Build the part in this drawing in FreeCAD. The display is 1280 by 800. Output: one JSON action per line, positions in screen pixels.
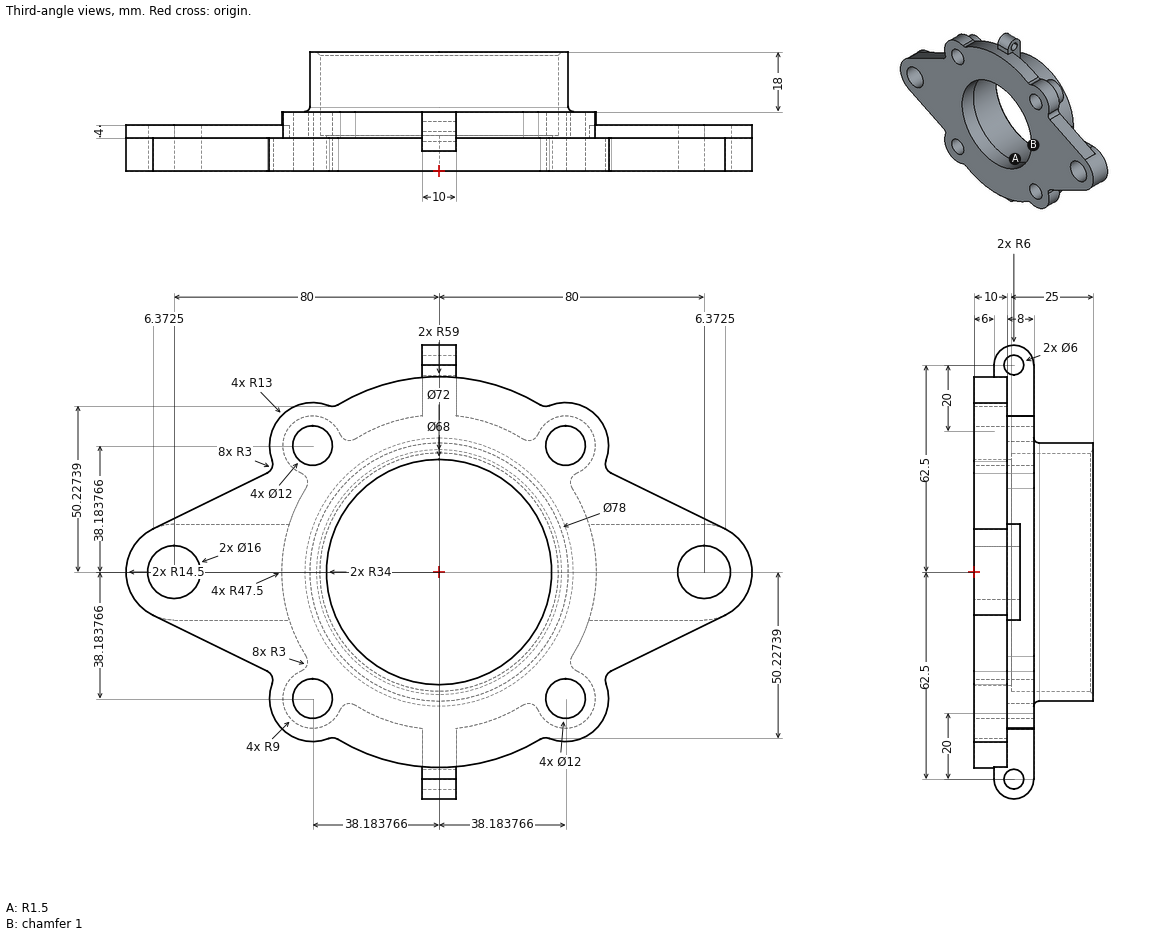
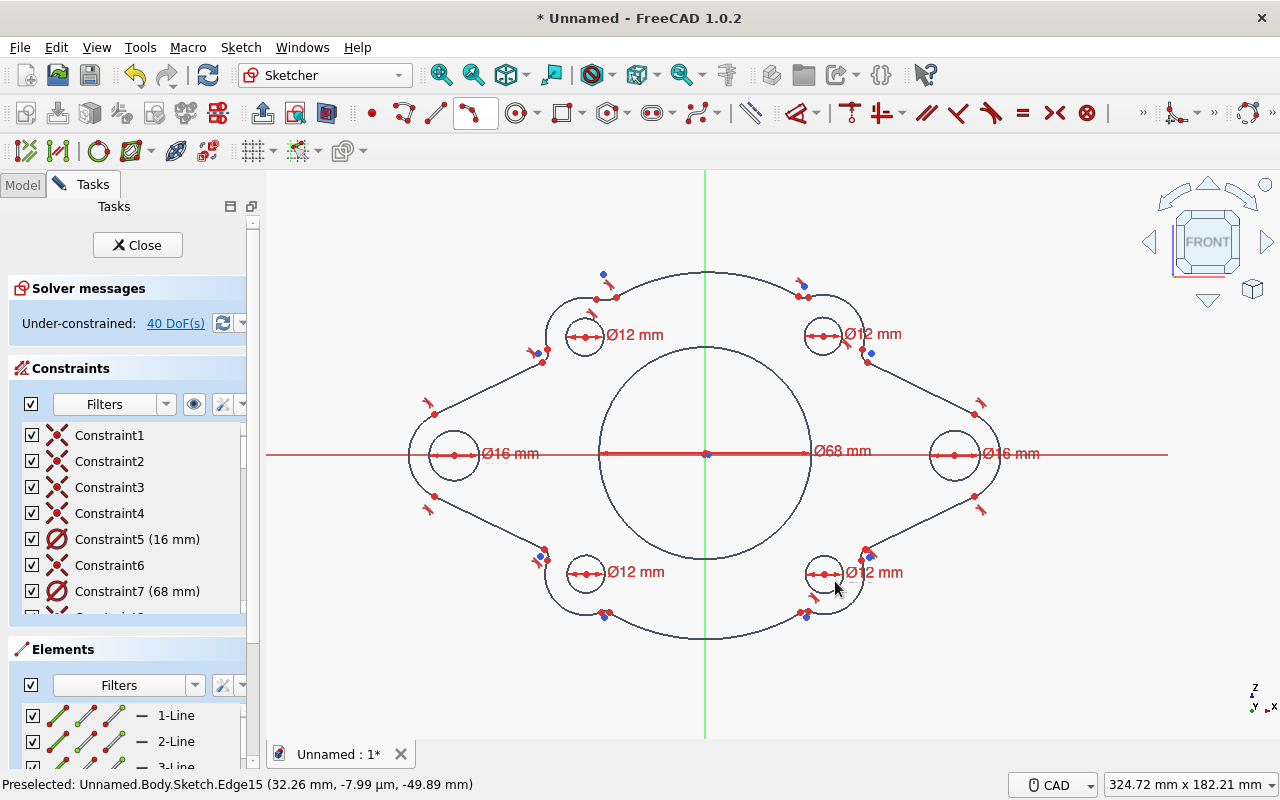
{"action": "left_click", "coordinate": [665, 635]}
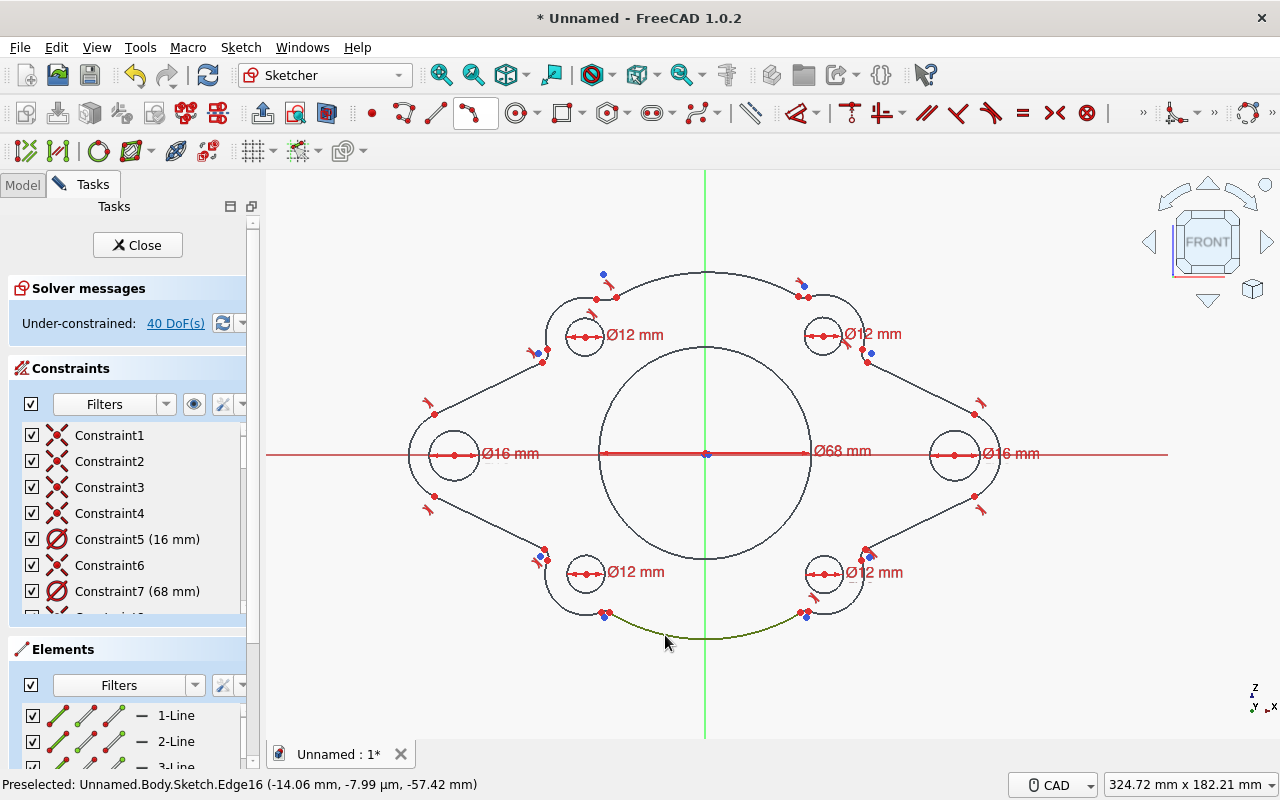
{"action": "left_click", "coordinate": [992, 114]}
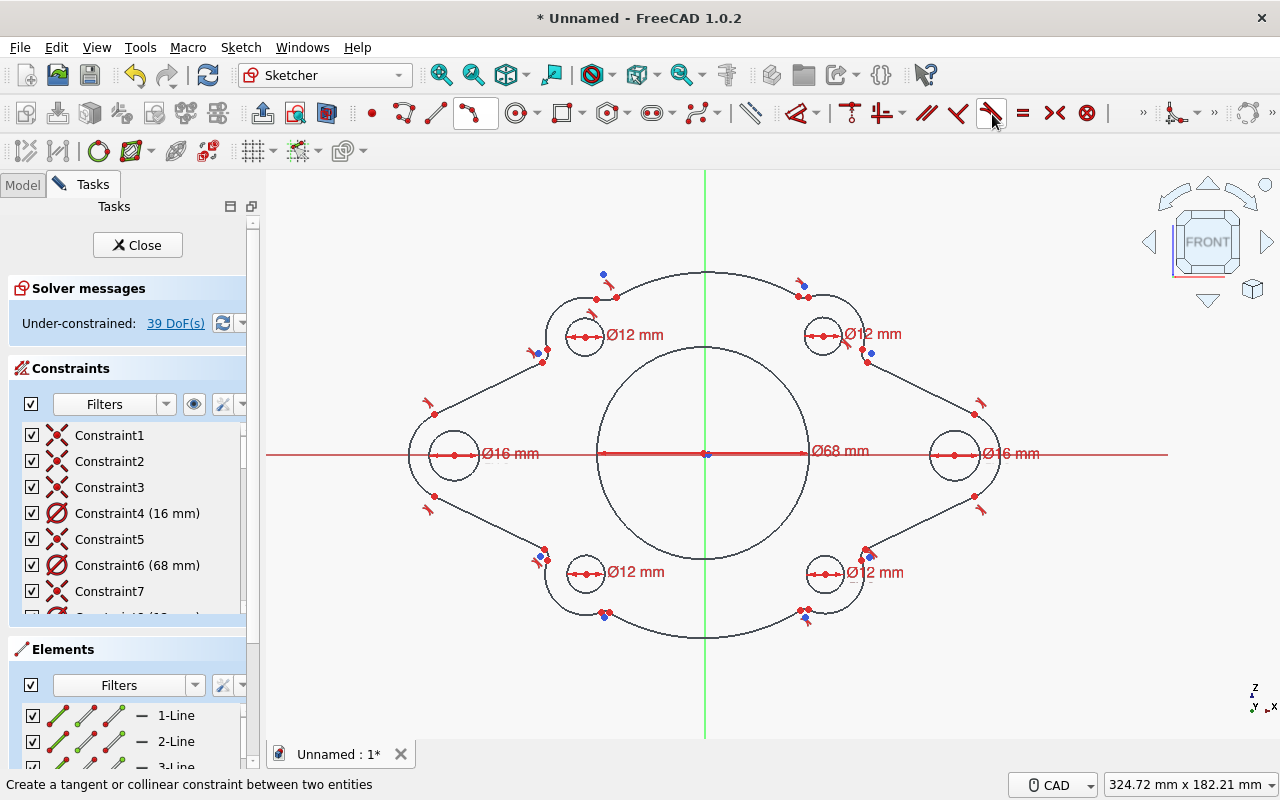
{"action": "left_click", "coordinate": [665, 634]}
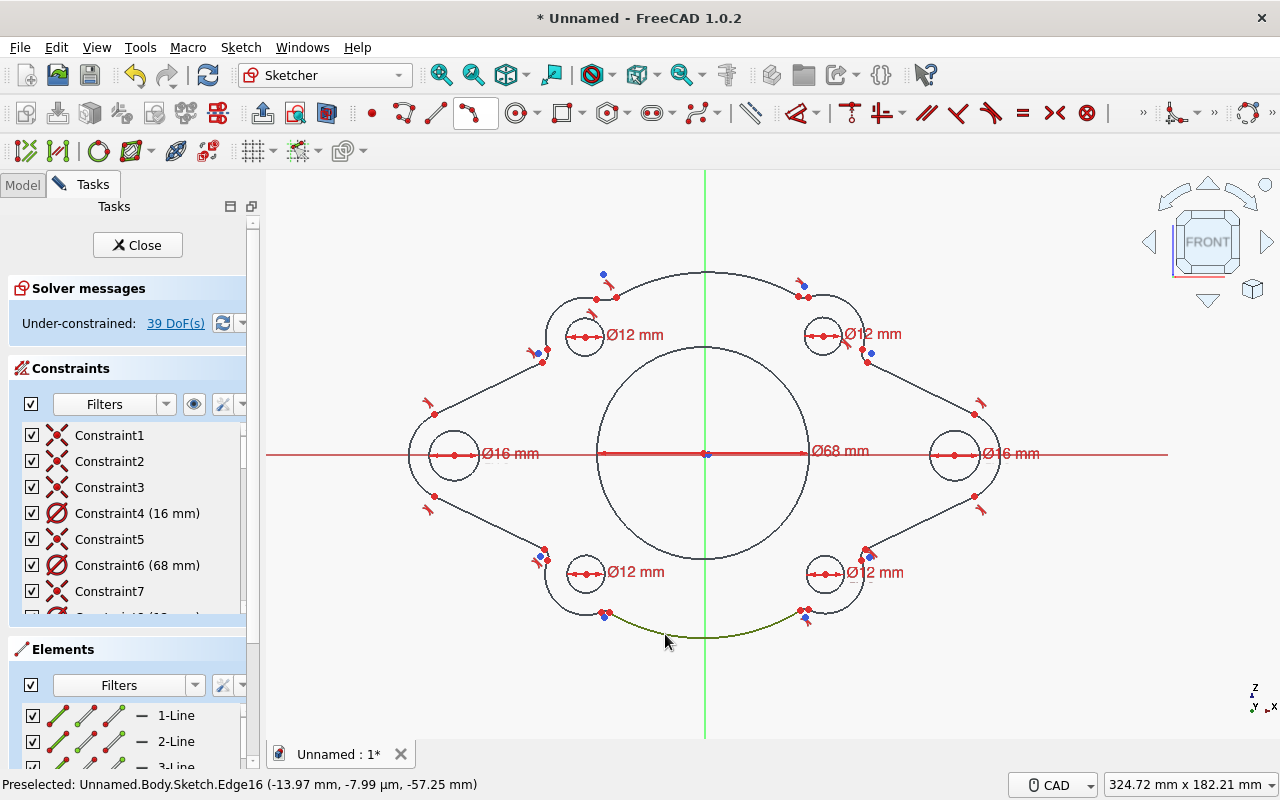
{"action": "scroll", "coordinate": [605, 611], "scroll_direction": "up", "scroll_amount": 6}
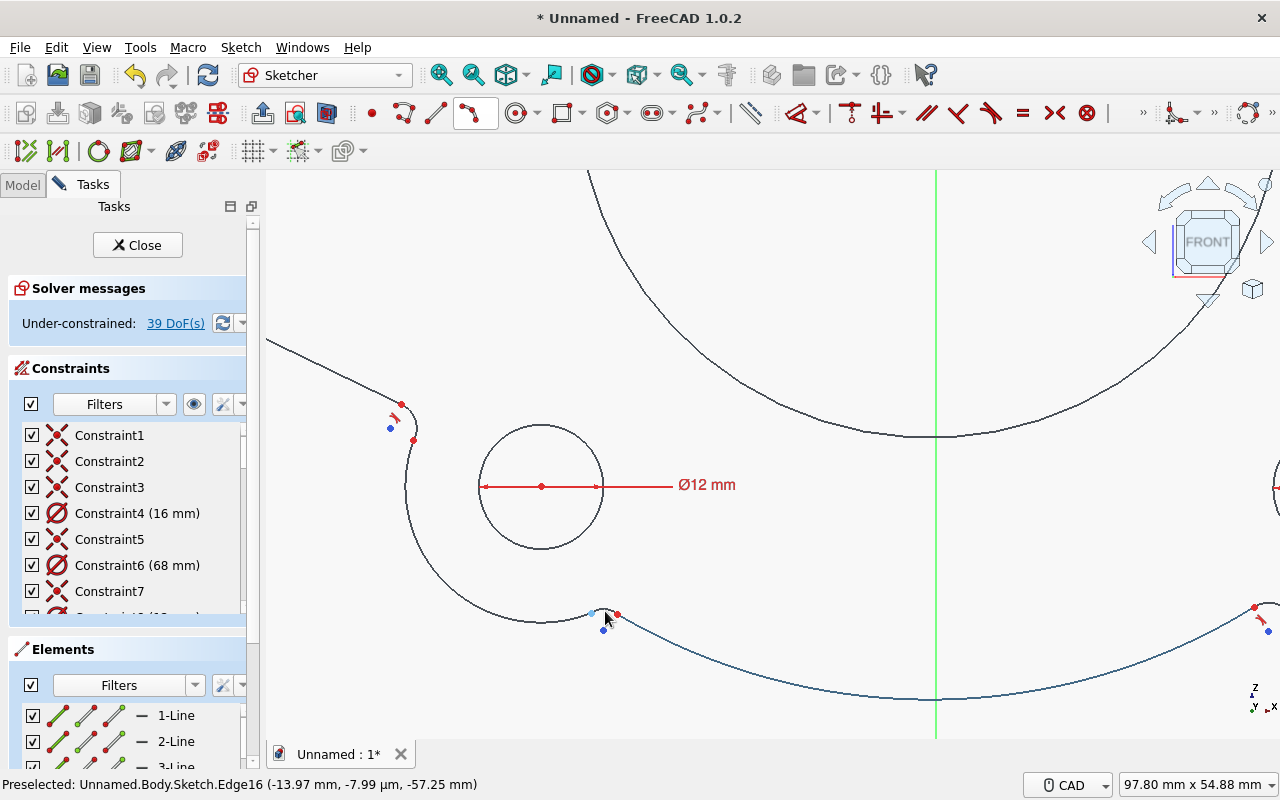
{"action": "left_click", "coordinate": [605, 609]}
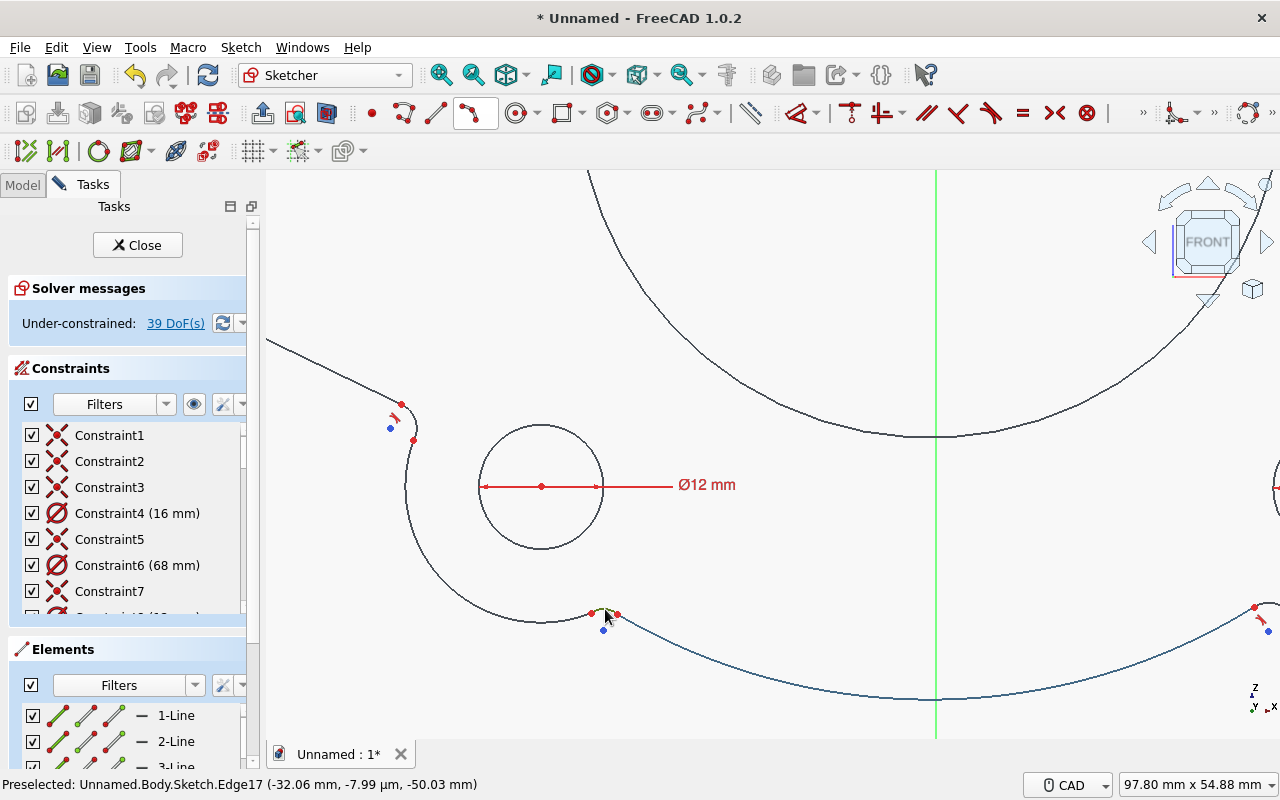
{"action": "left_click", "coordinate": [992, 114]}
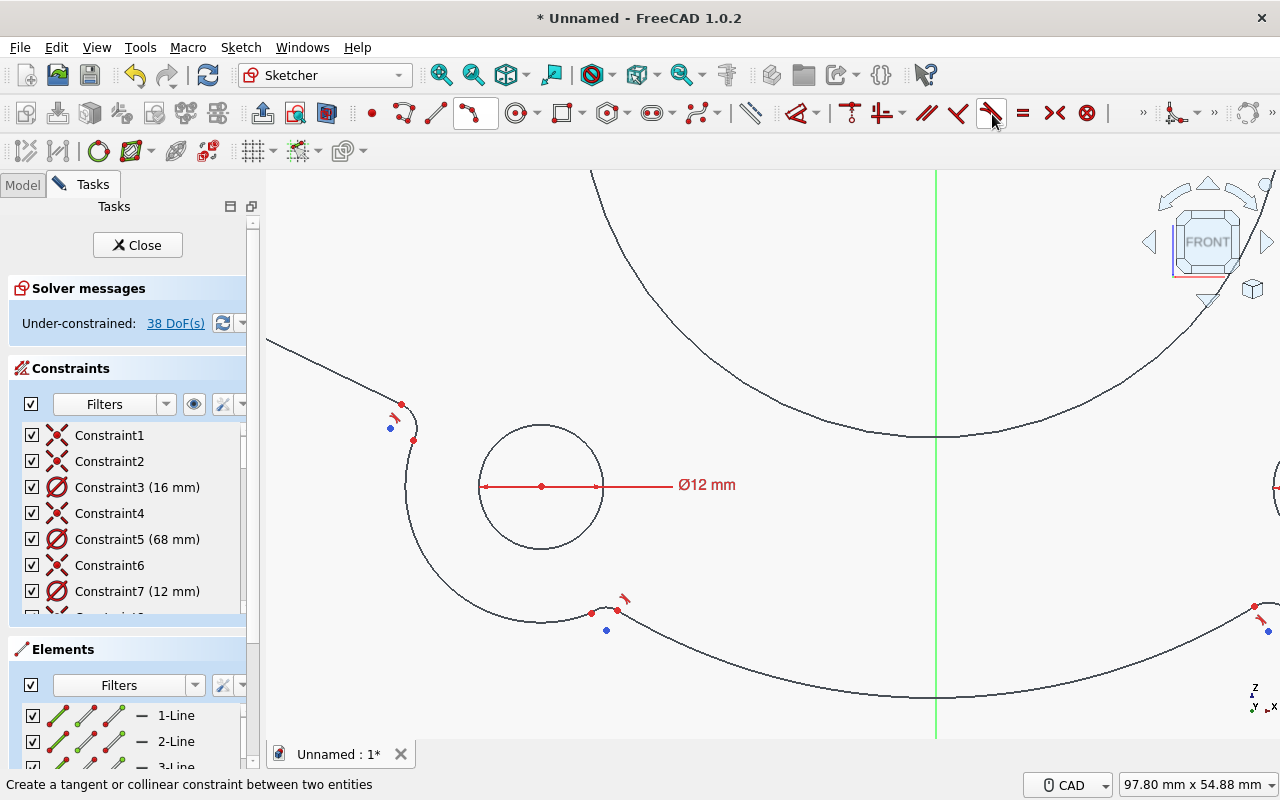
{"action": "left_click", "coordinate": [604, 608]}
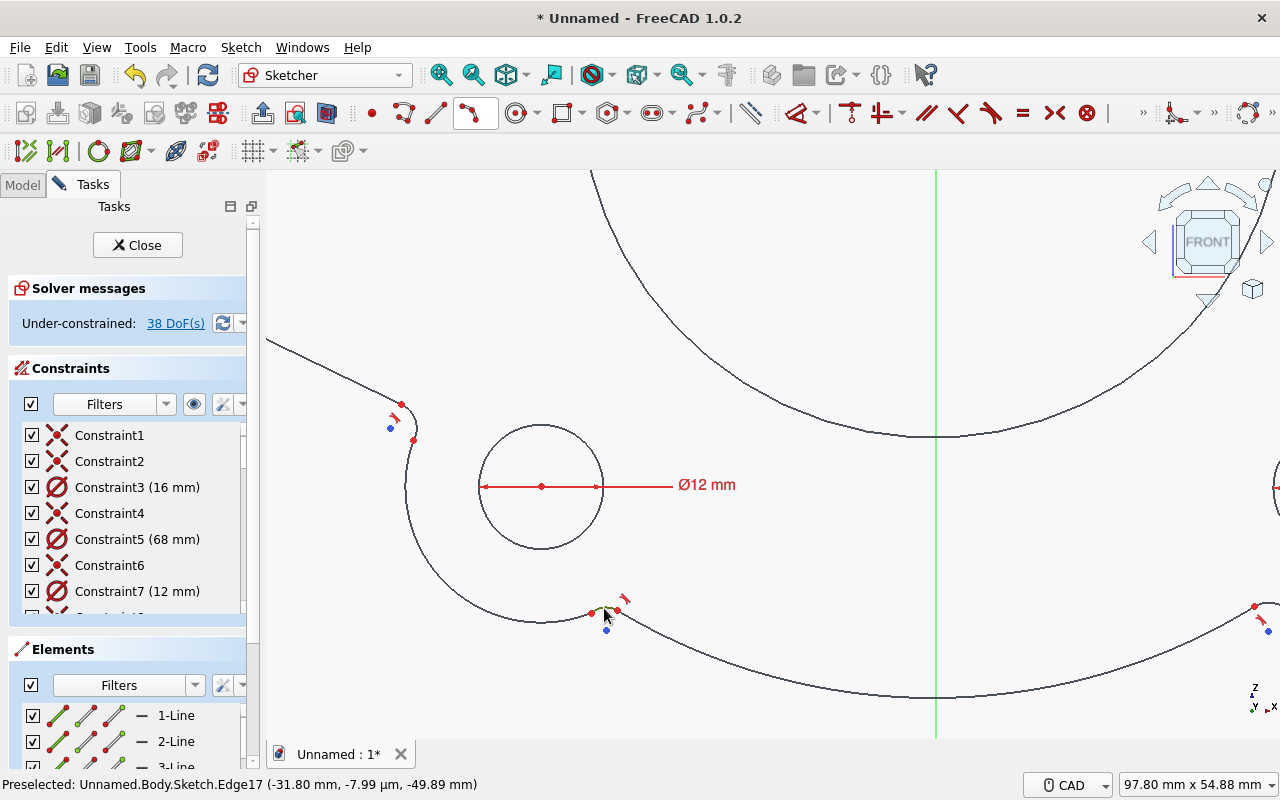
{"action": "left_click", "coordinate": [413, 532]}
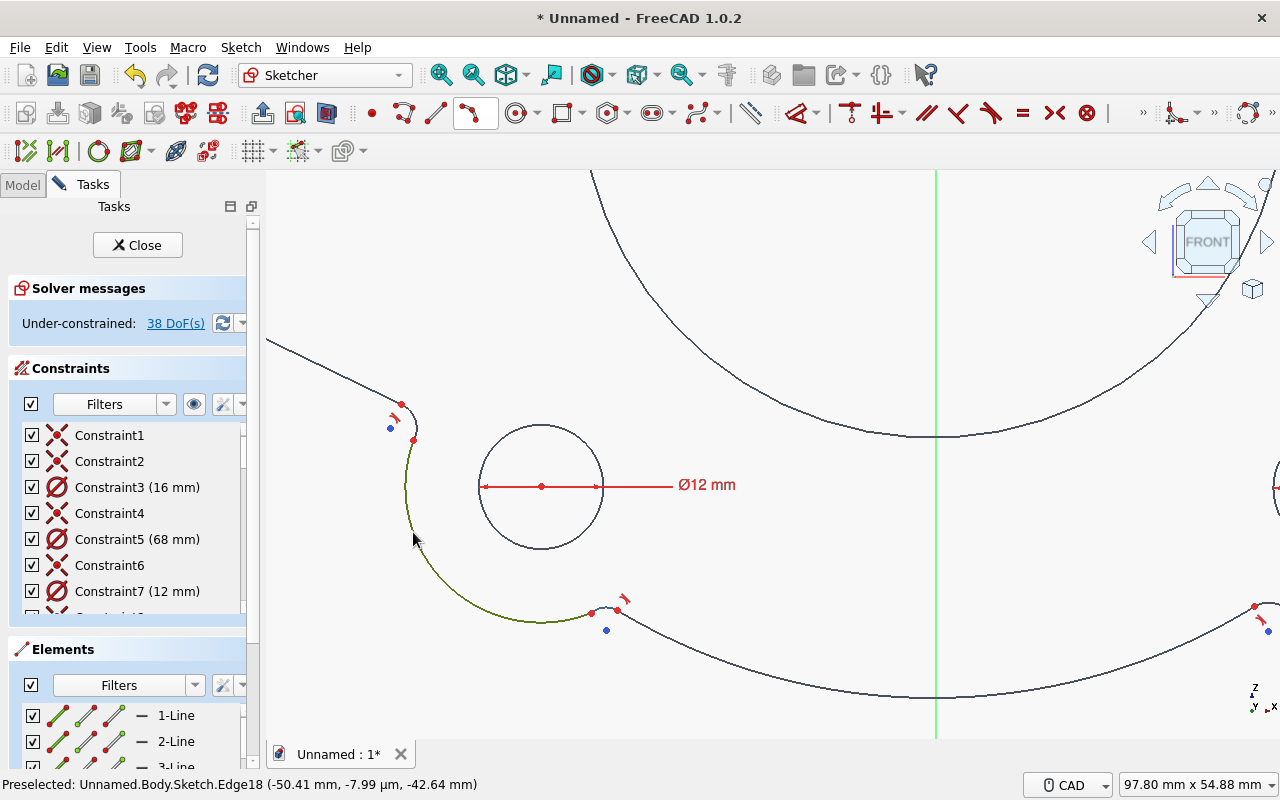
{"action": "left_click", "coordinate": [992, 114]}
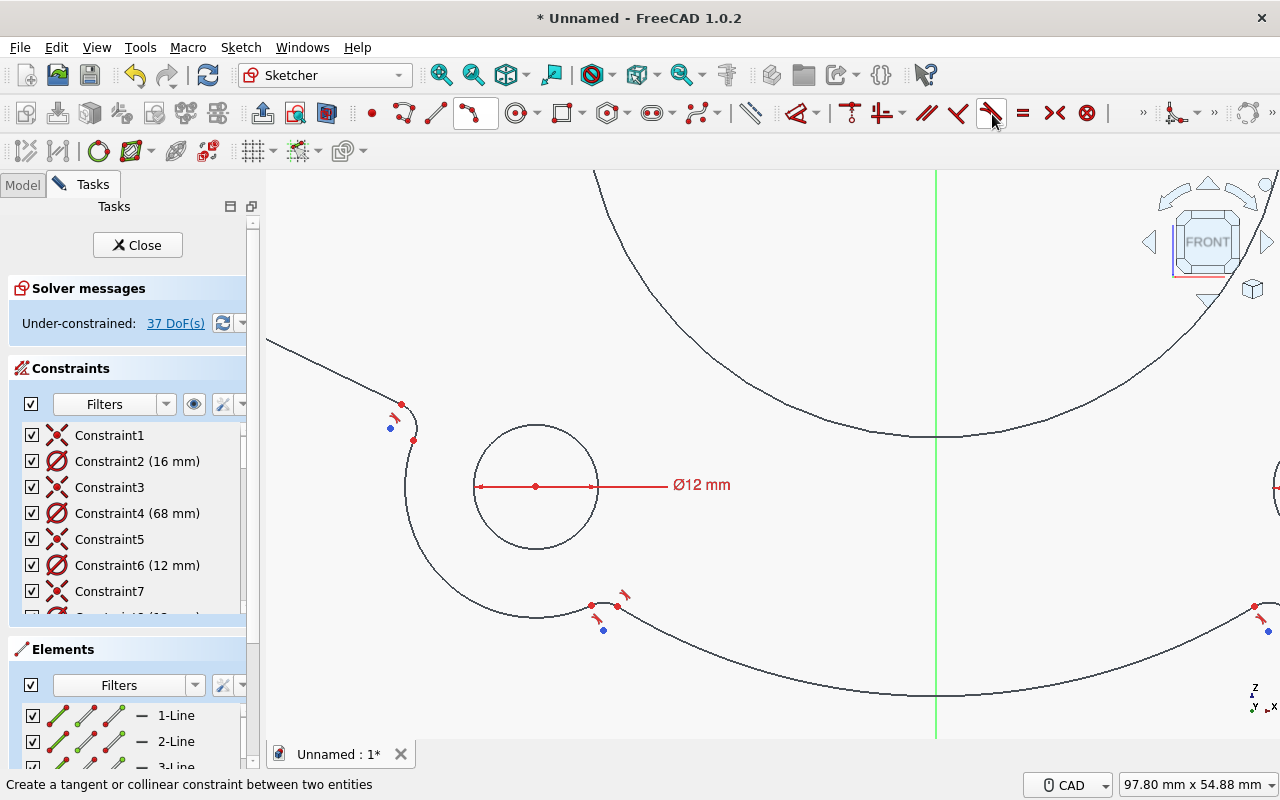
{"action": "left_click", "coordinate": [413, 532]}